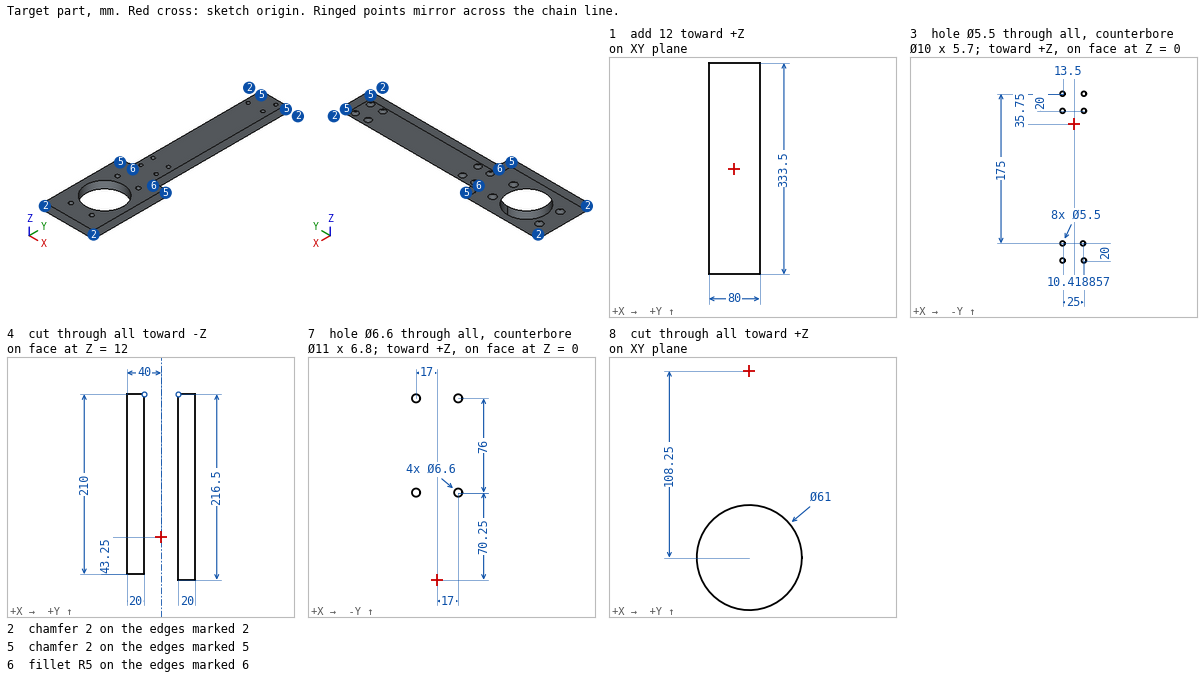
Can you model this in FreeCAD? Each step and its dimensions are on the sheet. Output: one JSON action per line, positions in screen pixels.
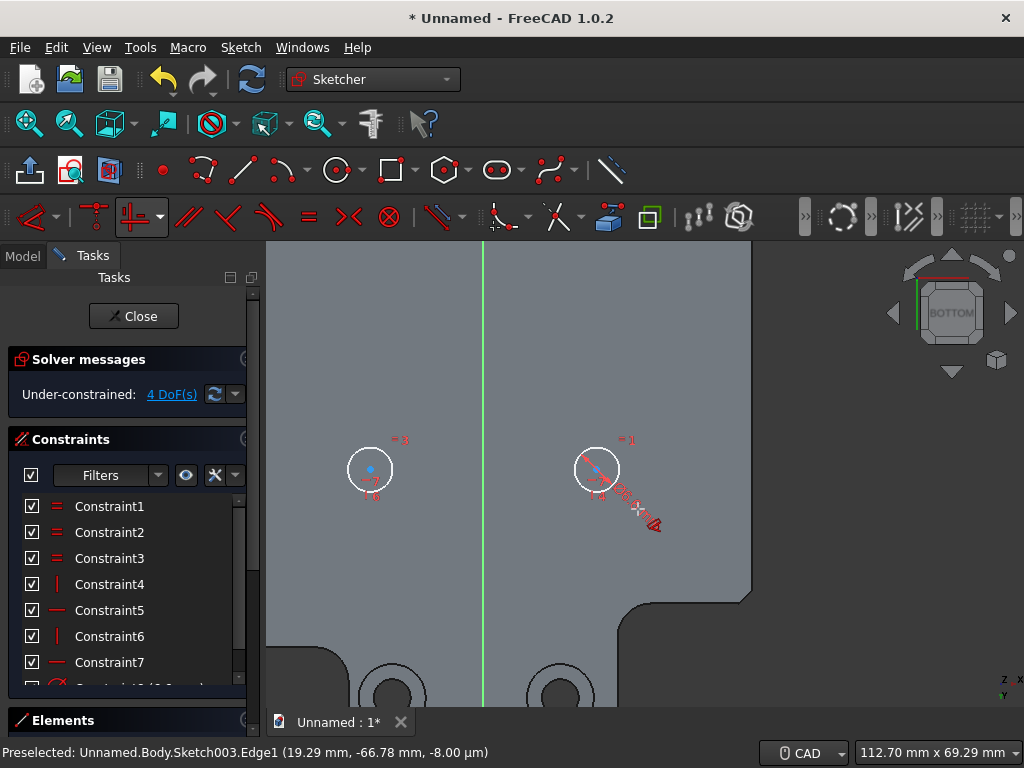
{"action": "left_click", "coordinate": [597, 470]}
{"action": "left_click", "coordinate": [540, 436]}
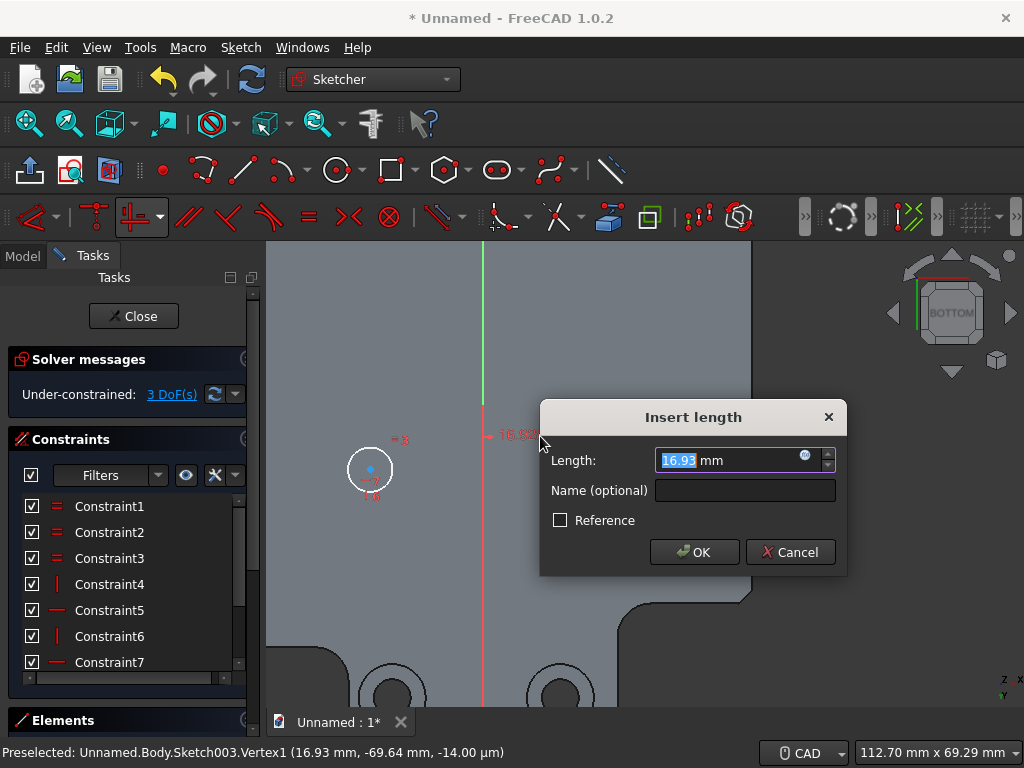
{"action": "type", "text": "17"}
{"action": "key", "text": "Return"}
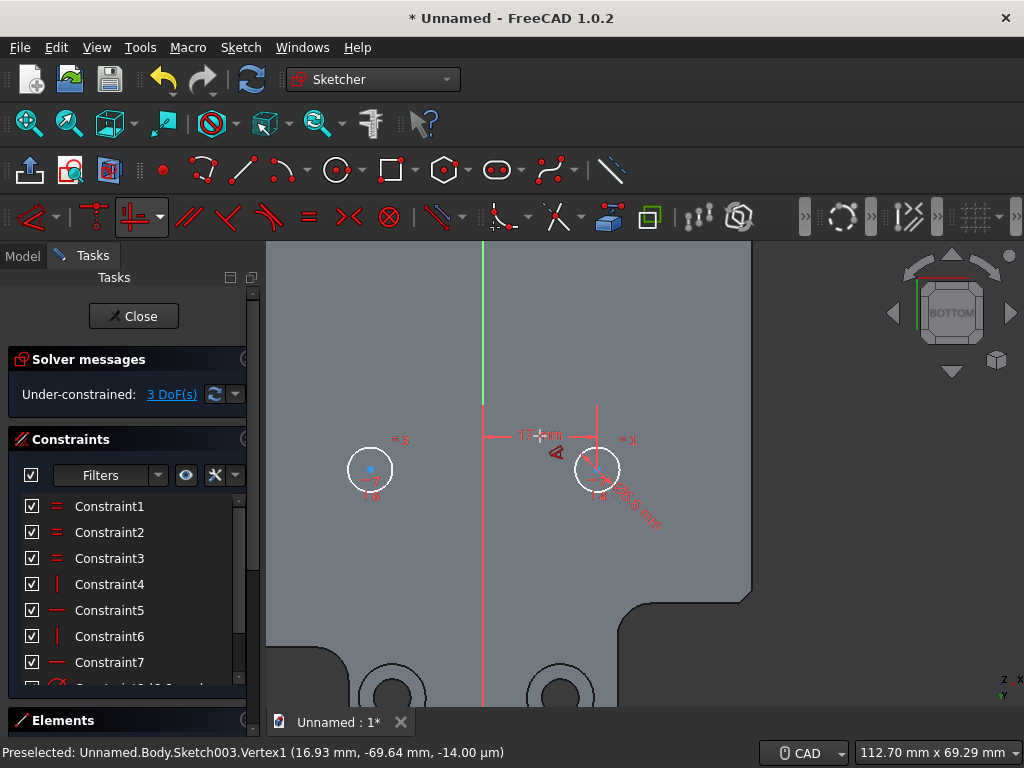
{"action": "scroll", "coordinate": [617, 491], "scroll_direction": "down", "scroll_amount": 6}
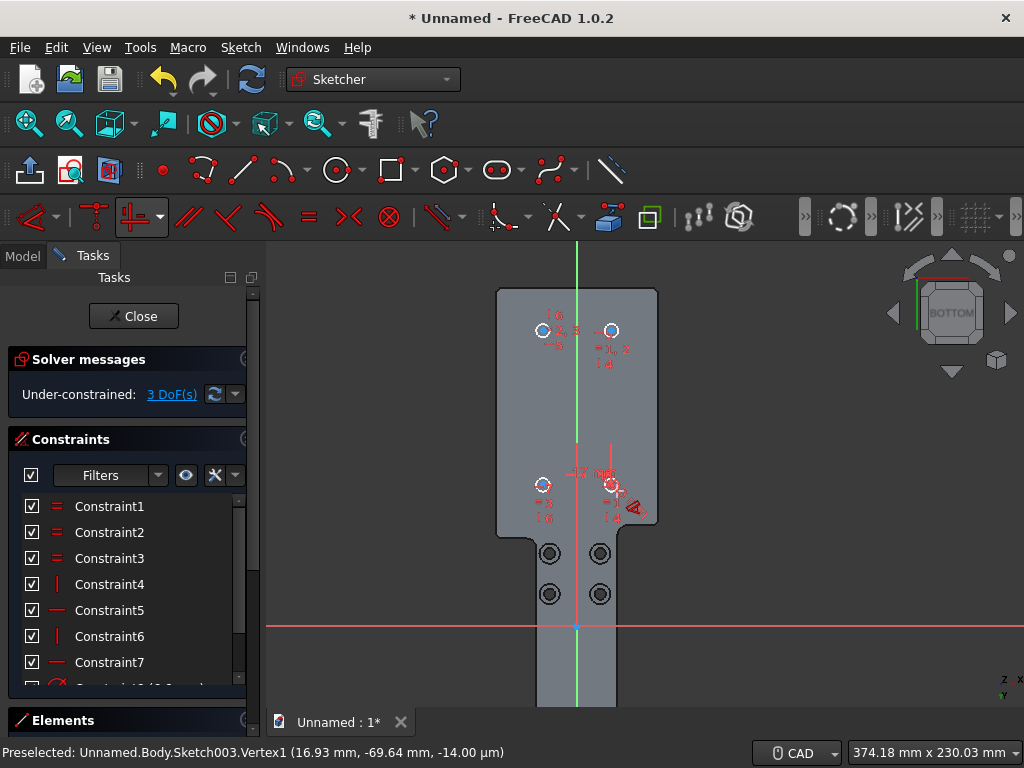
{"action": "left_click", "coordinate": [543, 331]}
{"action": "left_click", "coordinate": [560, 660]}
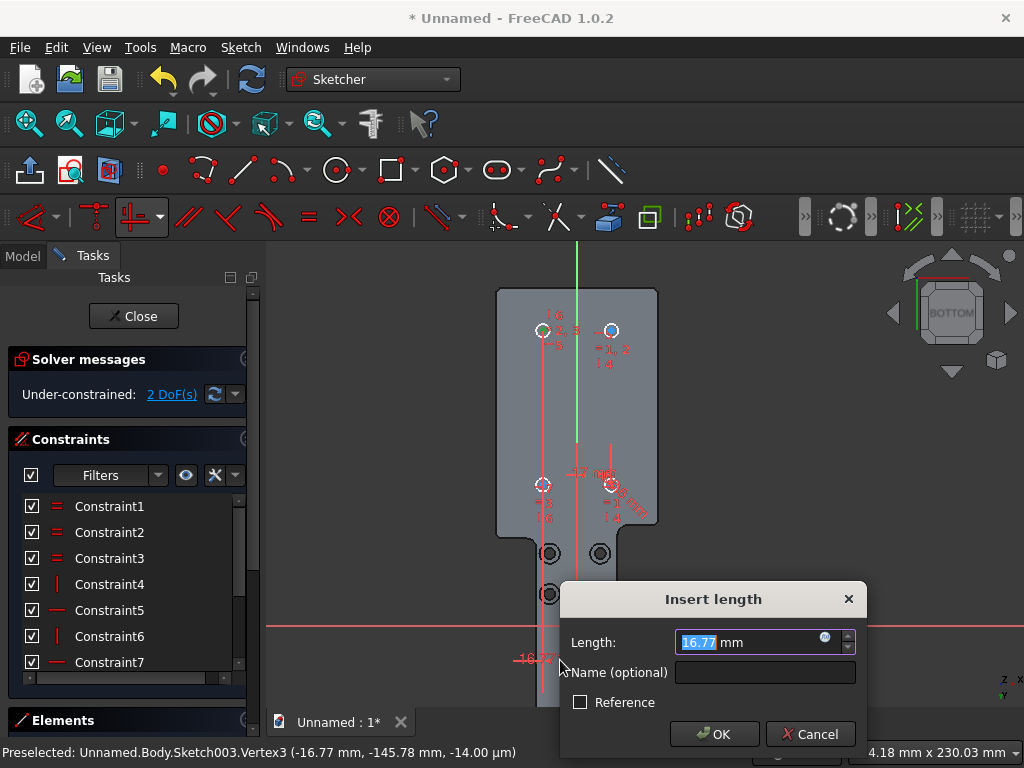
{"action": "type", "text": "17"}
{"action": "key", "text": "Return"}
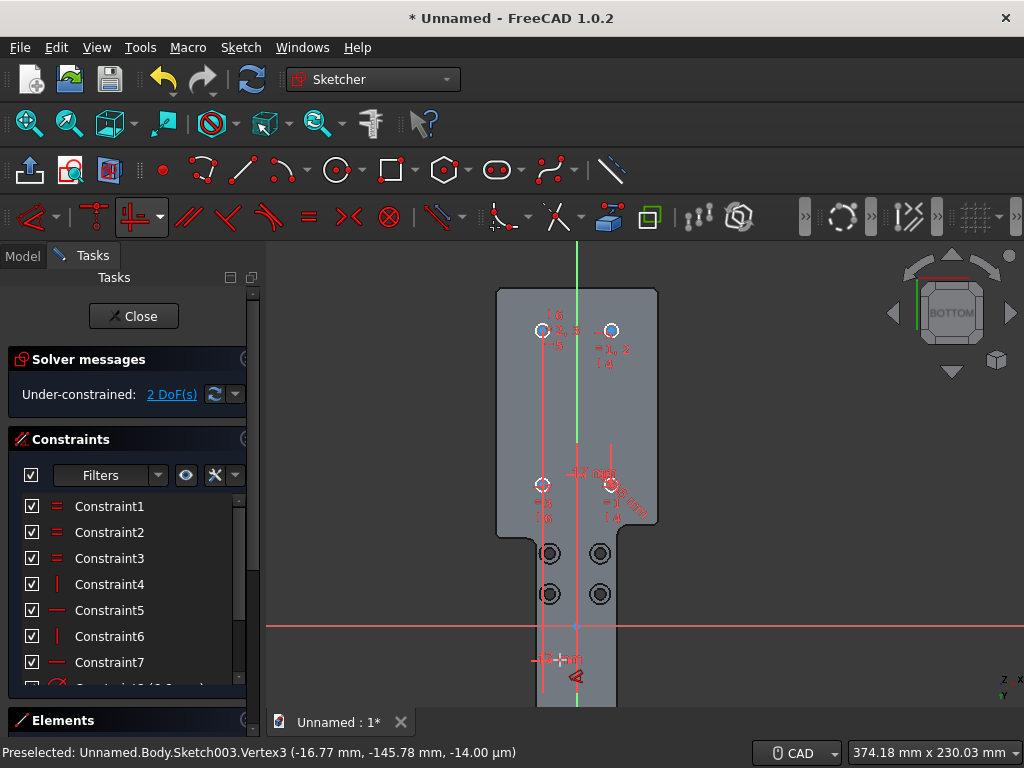
{"action": "left_click", "coordinate": [611, 485]}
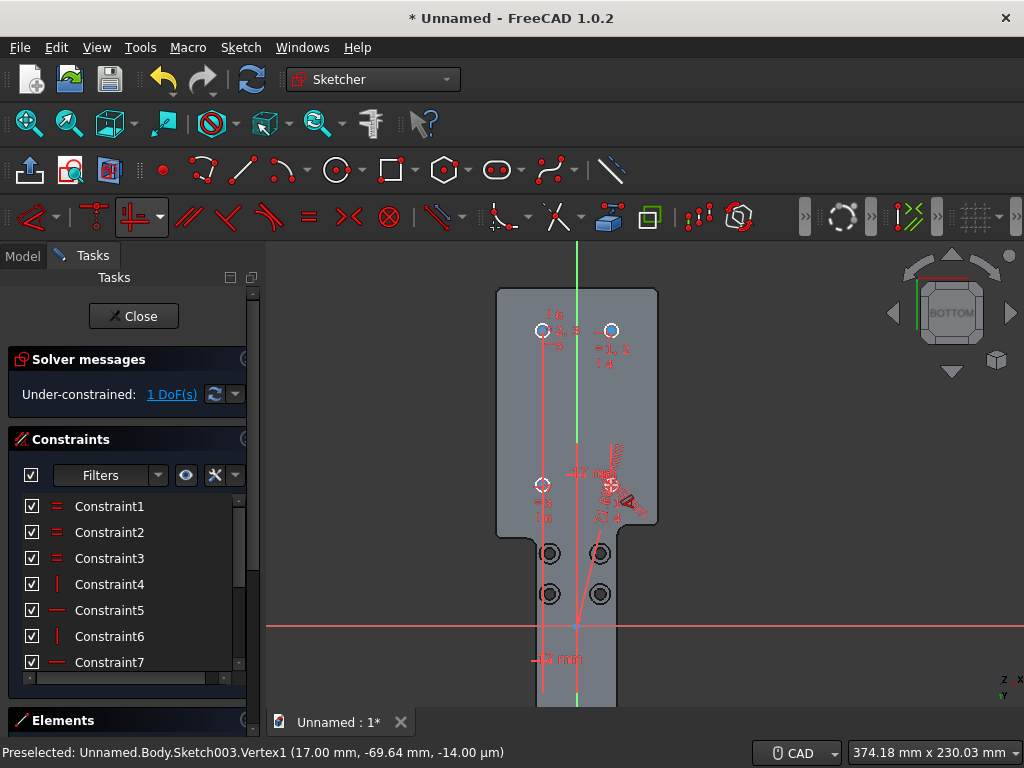
{"action": "left_click", "coordinate": [611, 331]}
{"action": "left_click", "coordinate": [645, 408]}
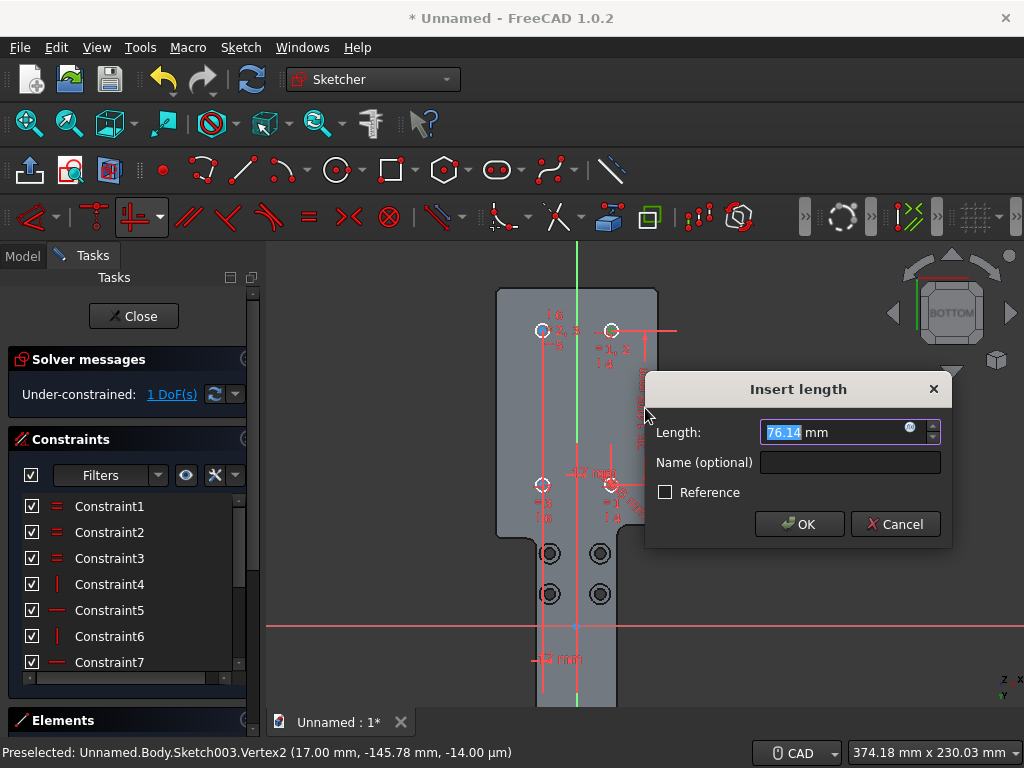
{"action": "type", "text": "76"}
{"action": "key", "text": "Return"}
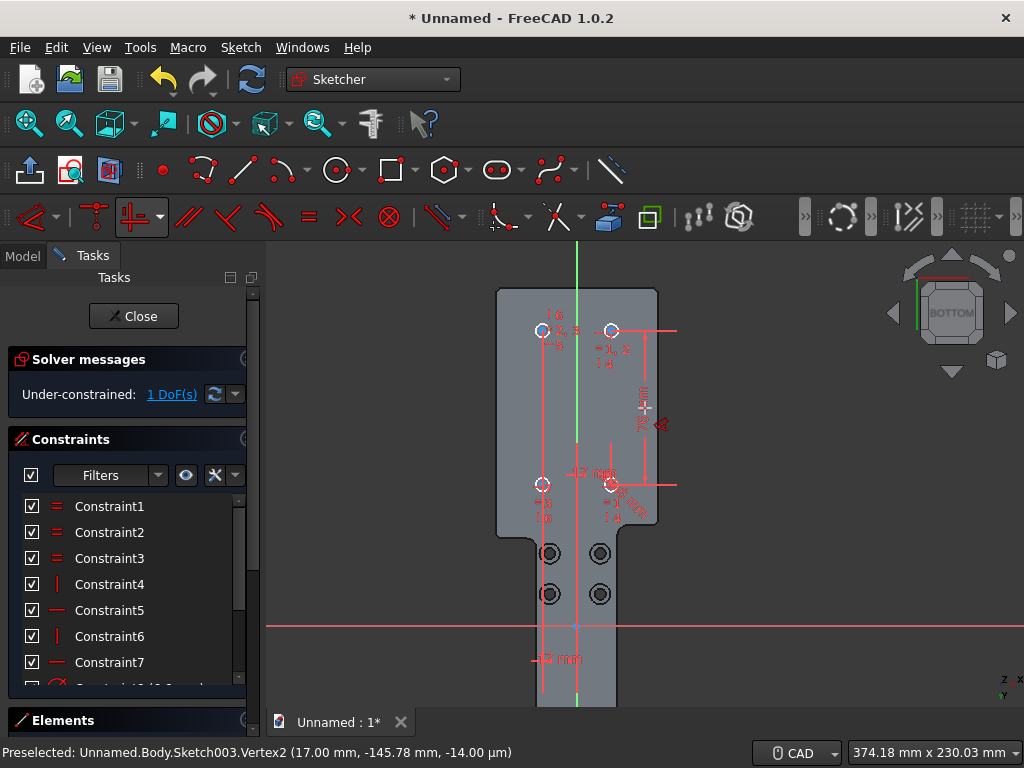
{"action": "left_click", "coordinate": [611, 485]}
{"action": "left_click", "coordinate": [645, 555]}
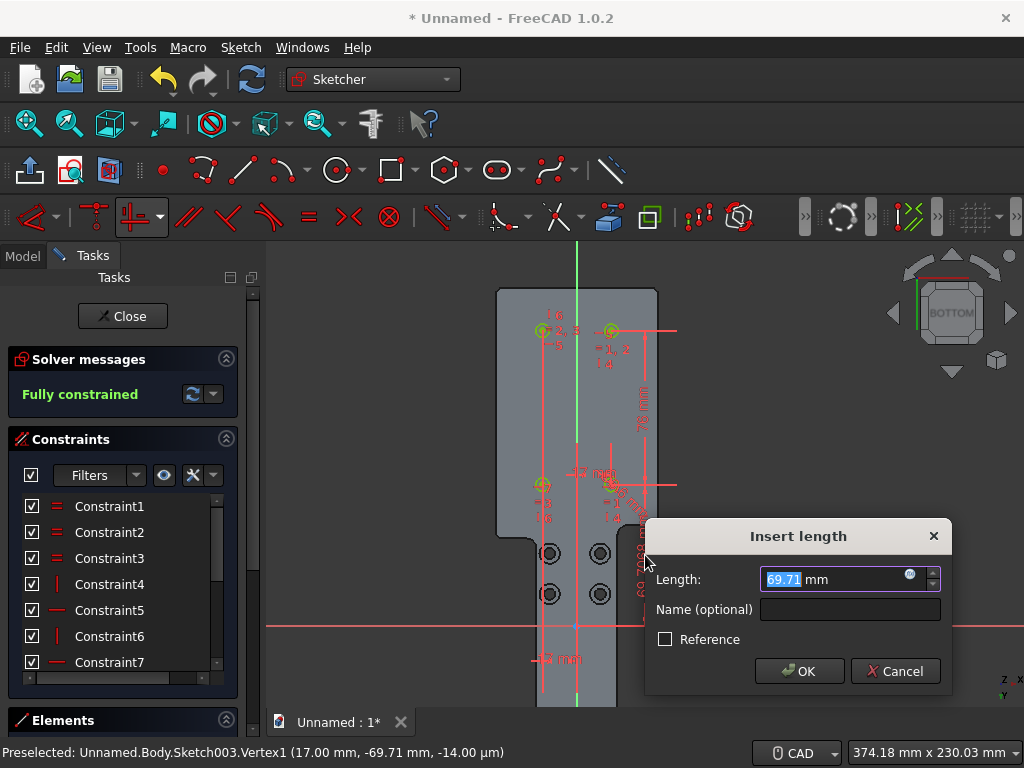
{"action": "type", "text": "70.25"}
{"action": "key", "text": "Return"}
{"action": "key", "text": "Escape"}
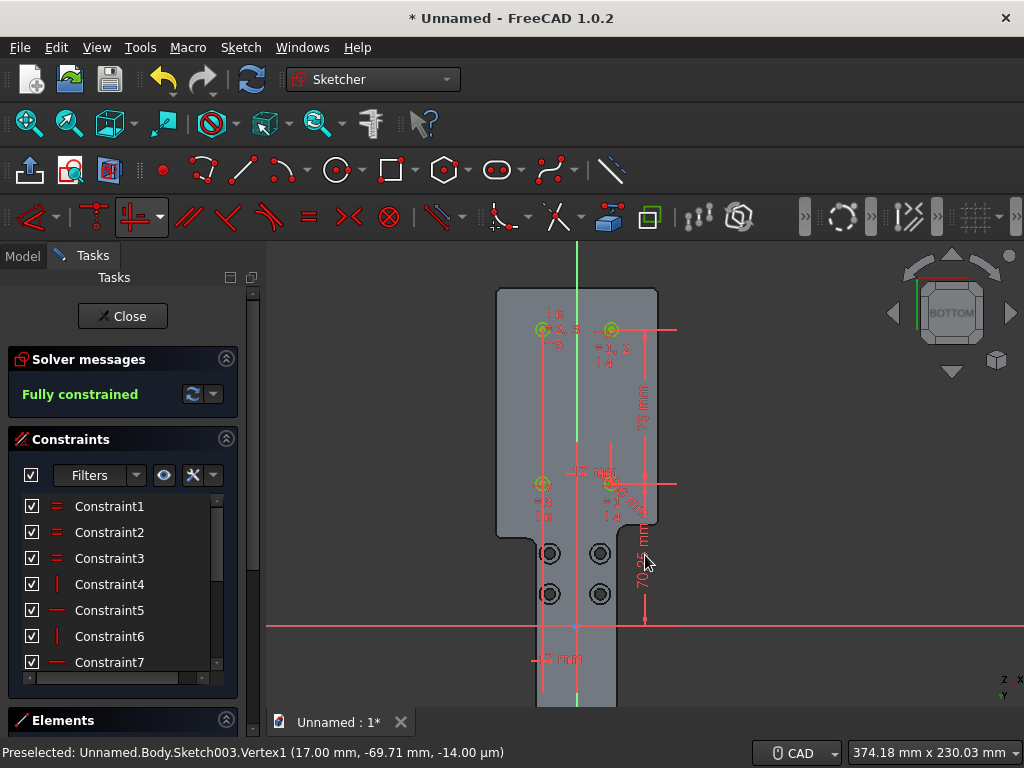
{"action": "left_click", "coordinate": [123, 316]}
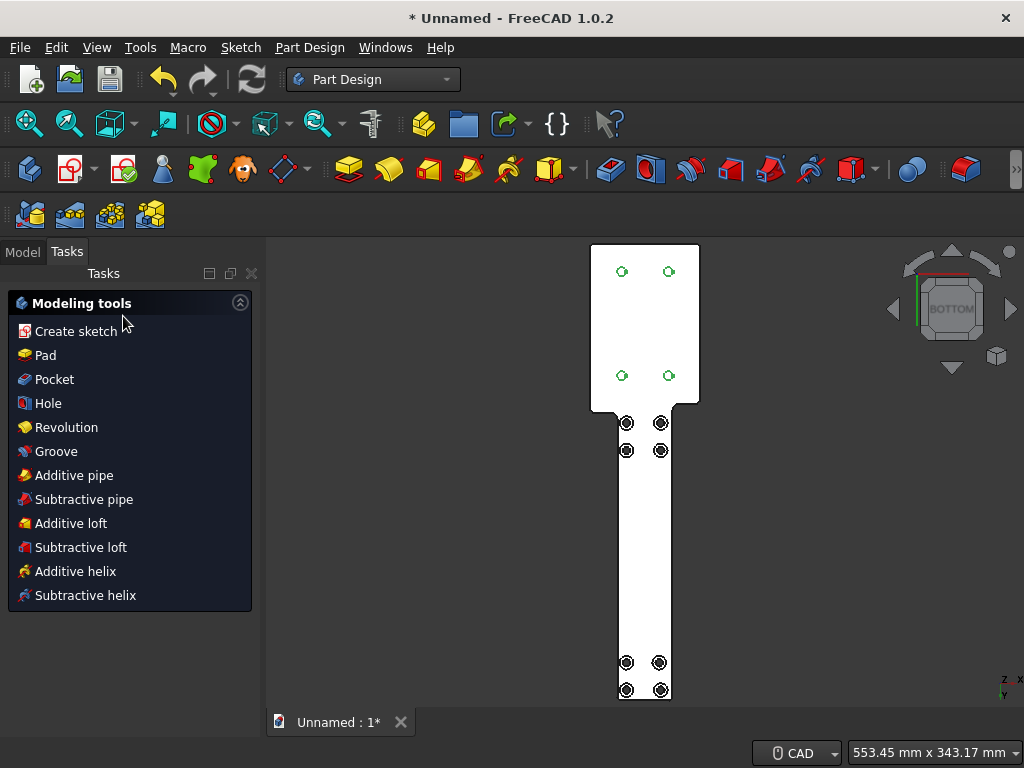
{"action": "left_click", "coordinate": [652, 170]}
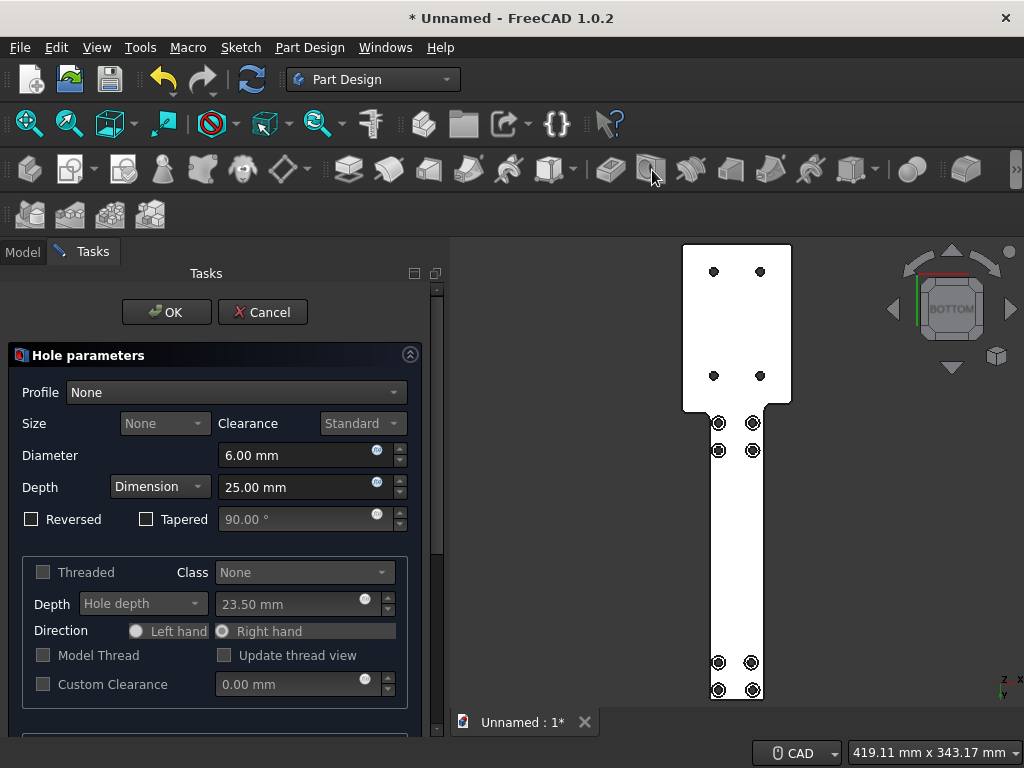
{"action": "triple_click", "coordinate": [305, 455]}